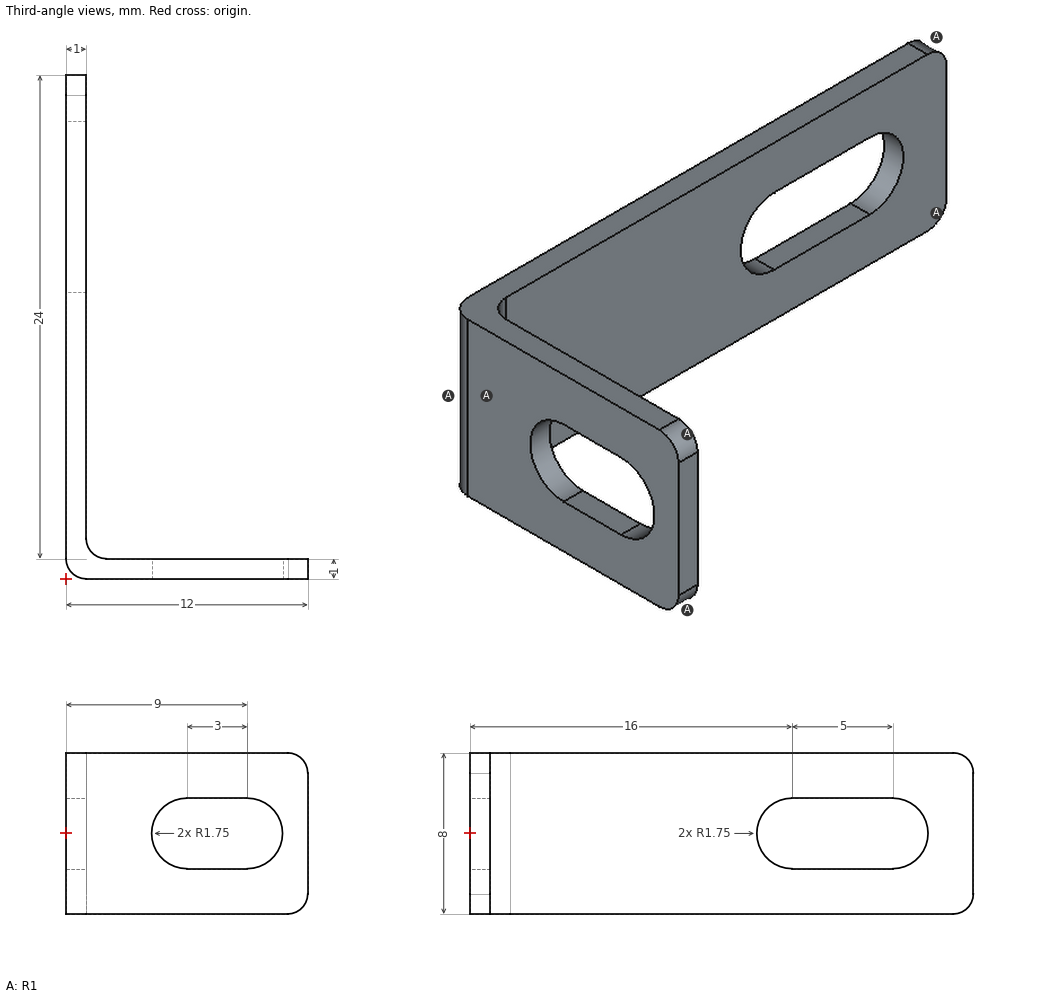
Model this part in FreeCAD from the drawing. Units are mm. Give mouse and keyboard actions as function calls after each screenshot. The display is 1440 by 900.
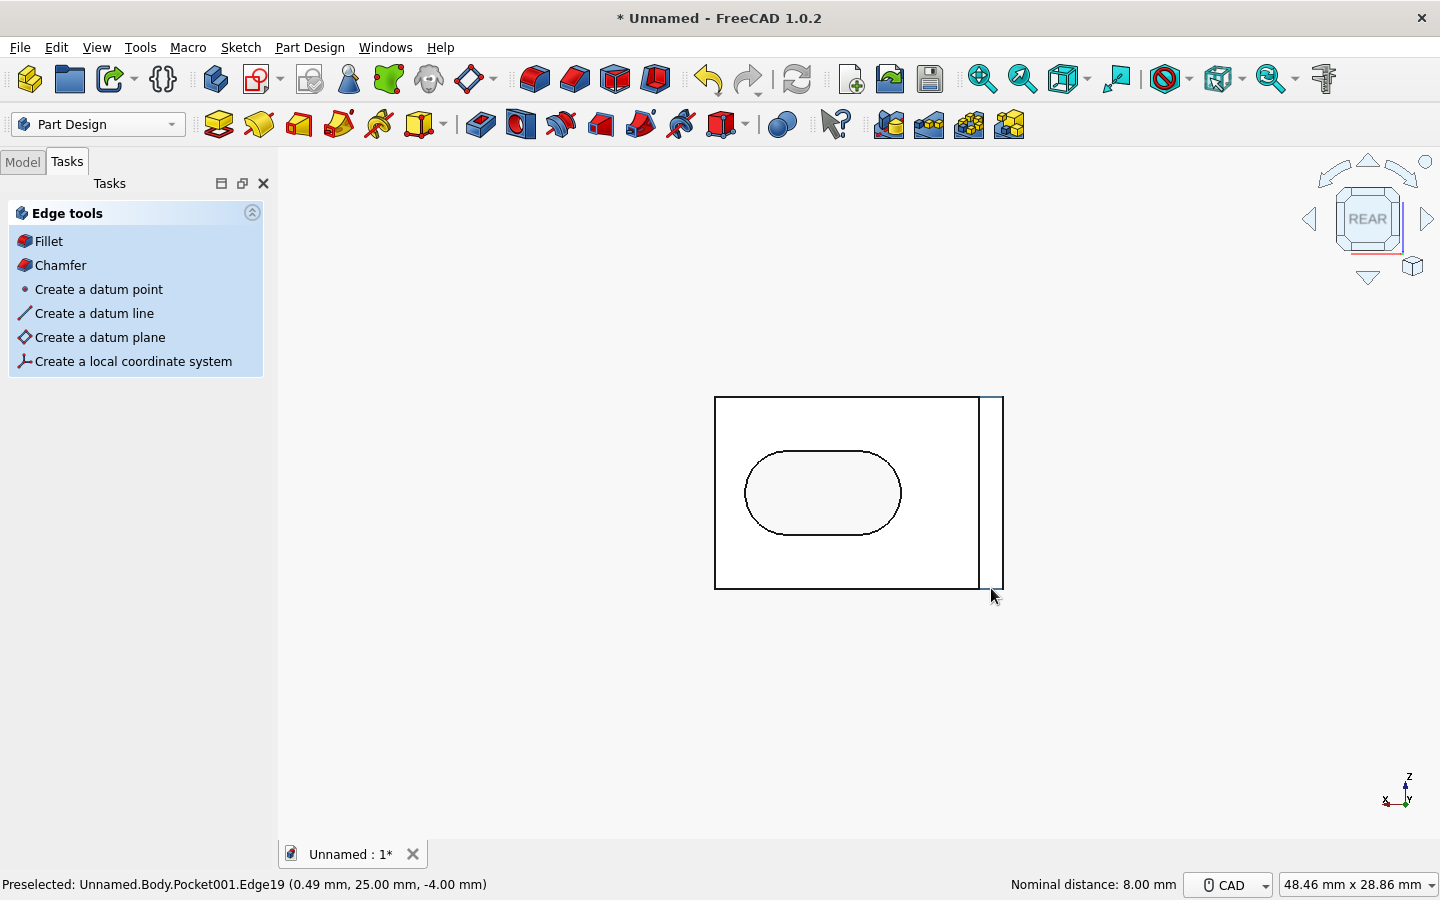
key(0)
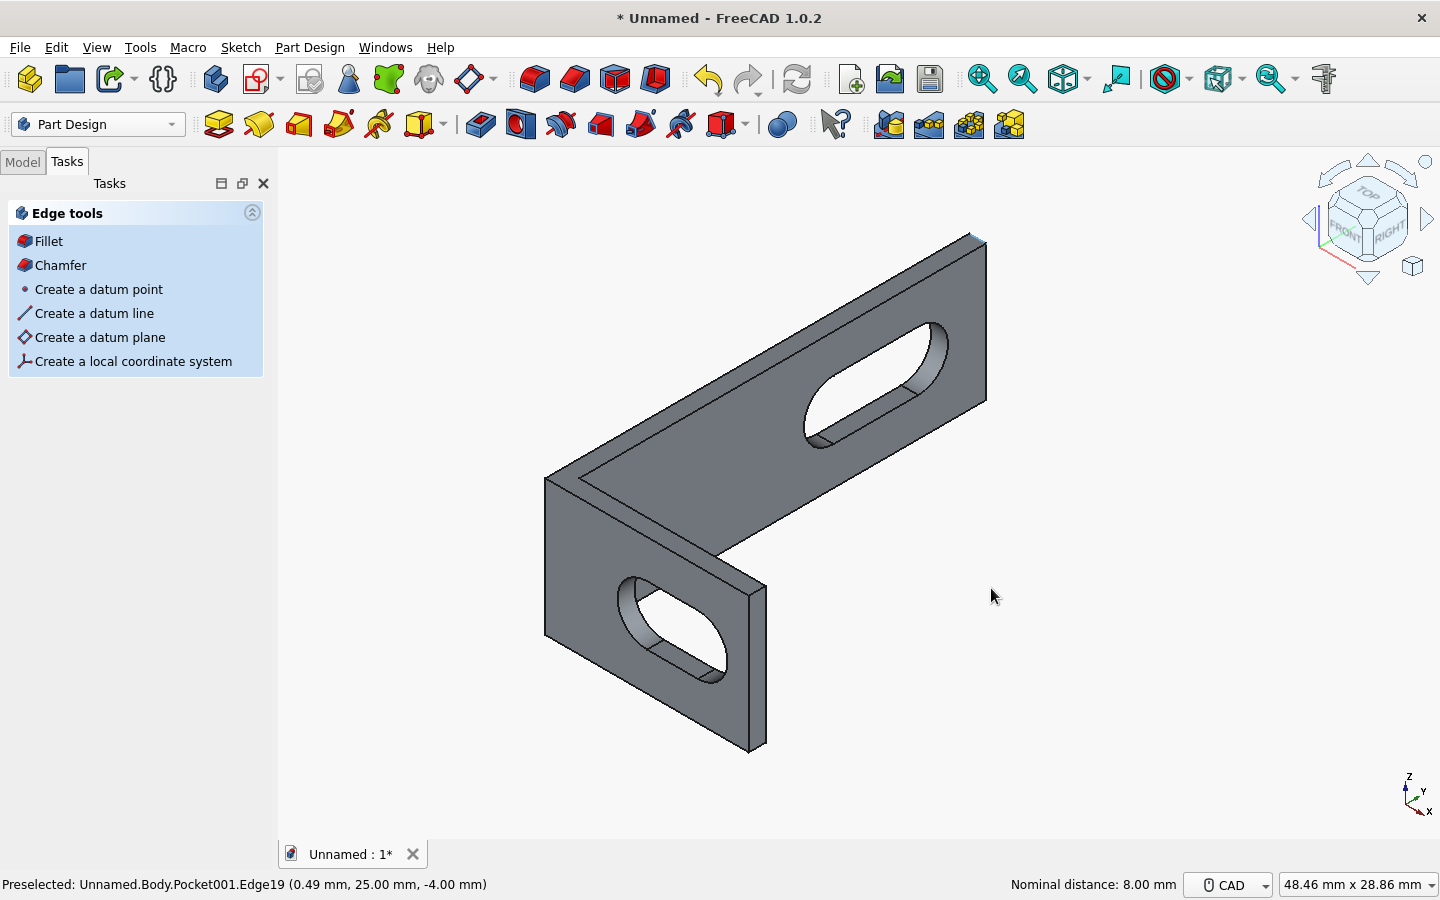
click(757, 590, ctrl)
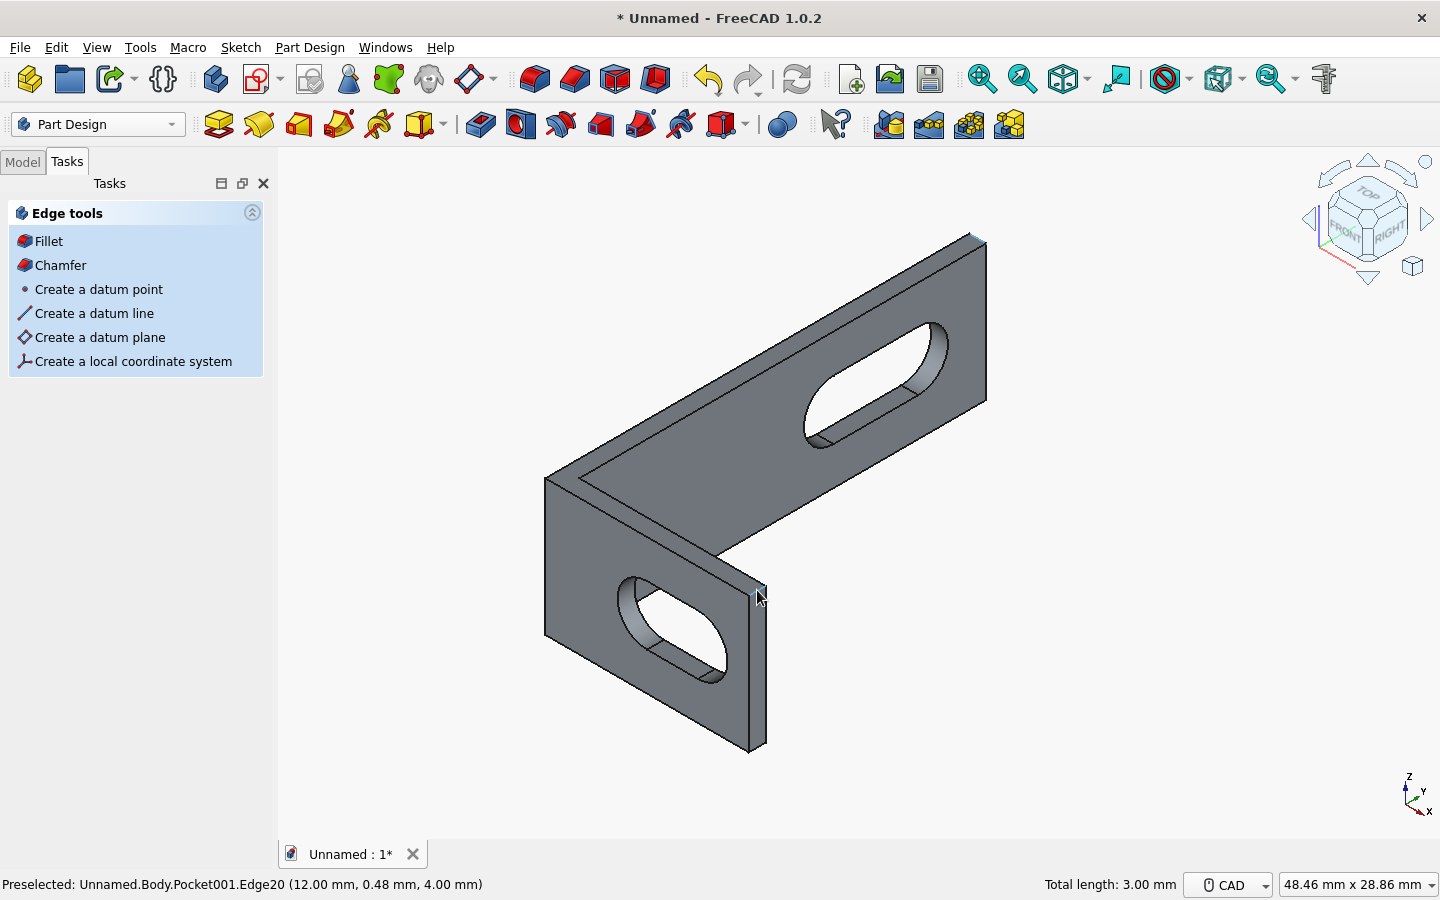
key(2)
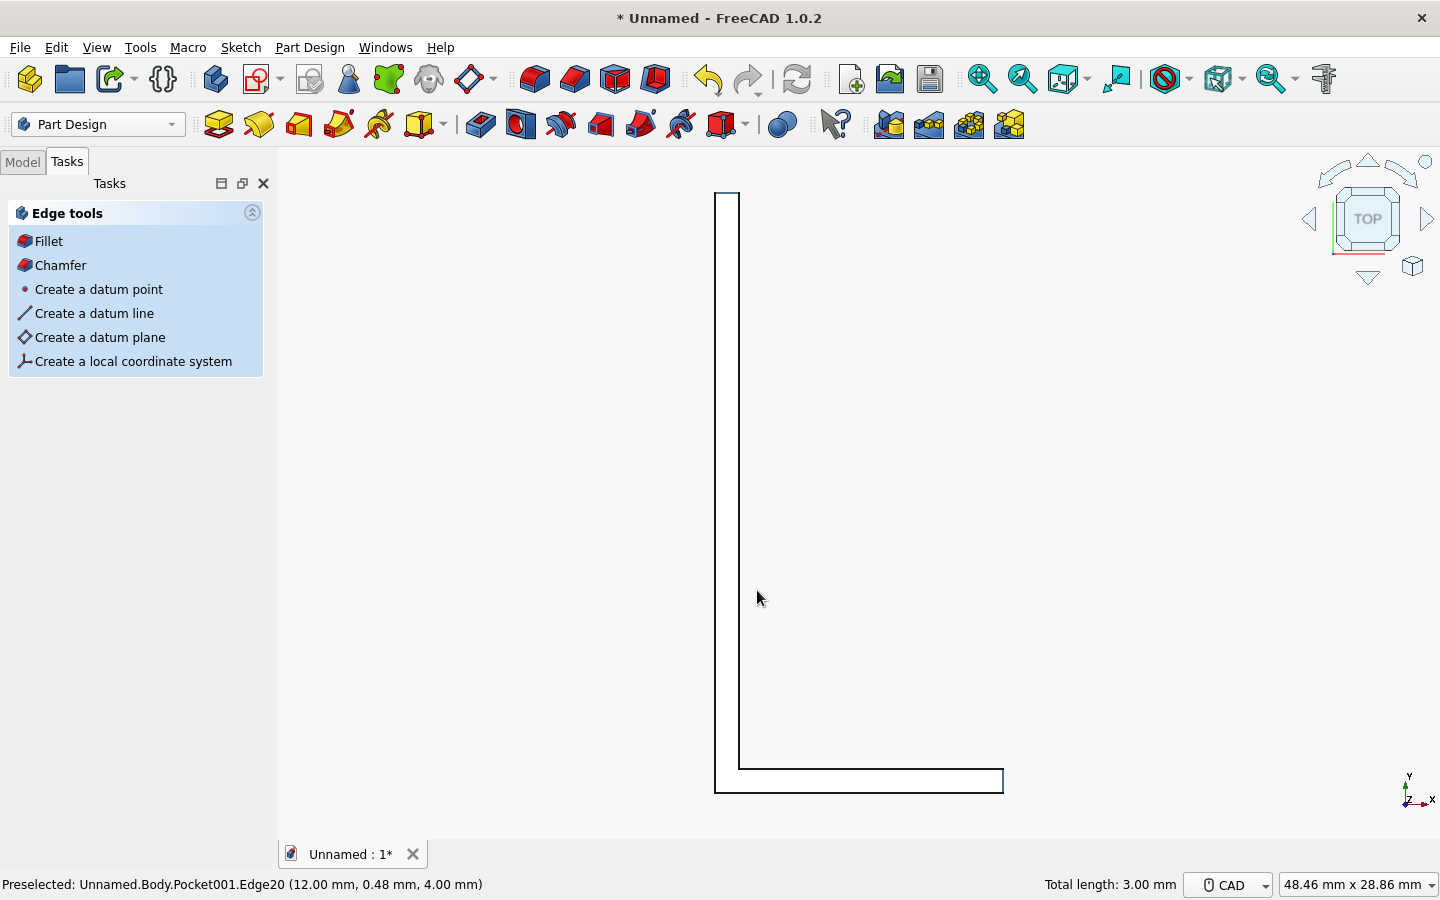
key(1)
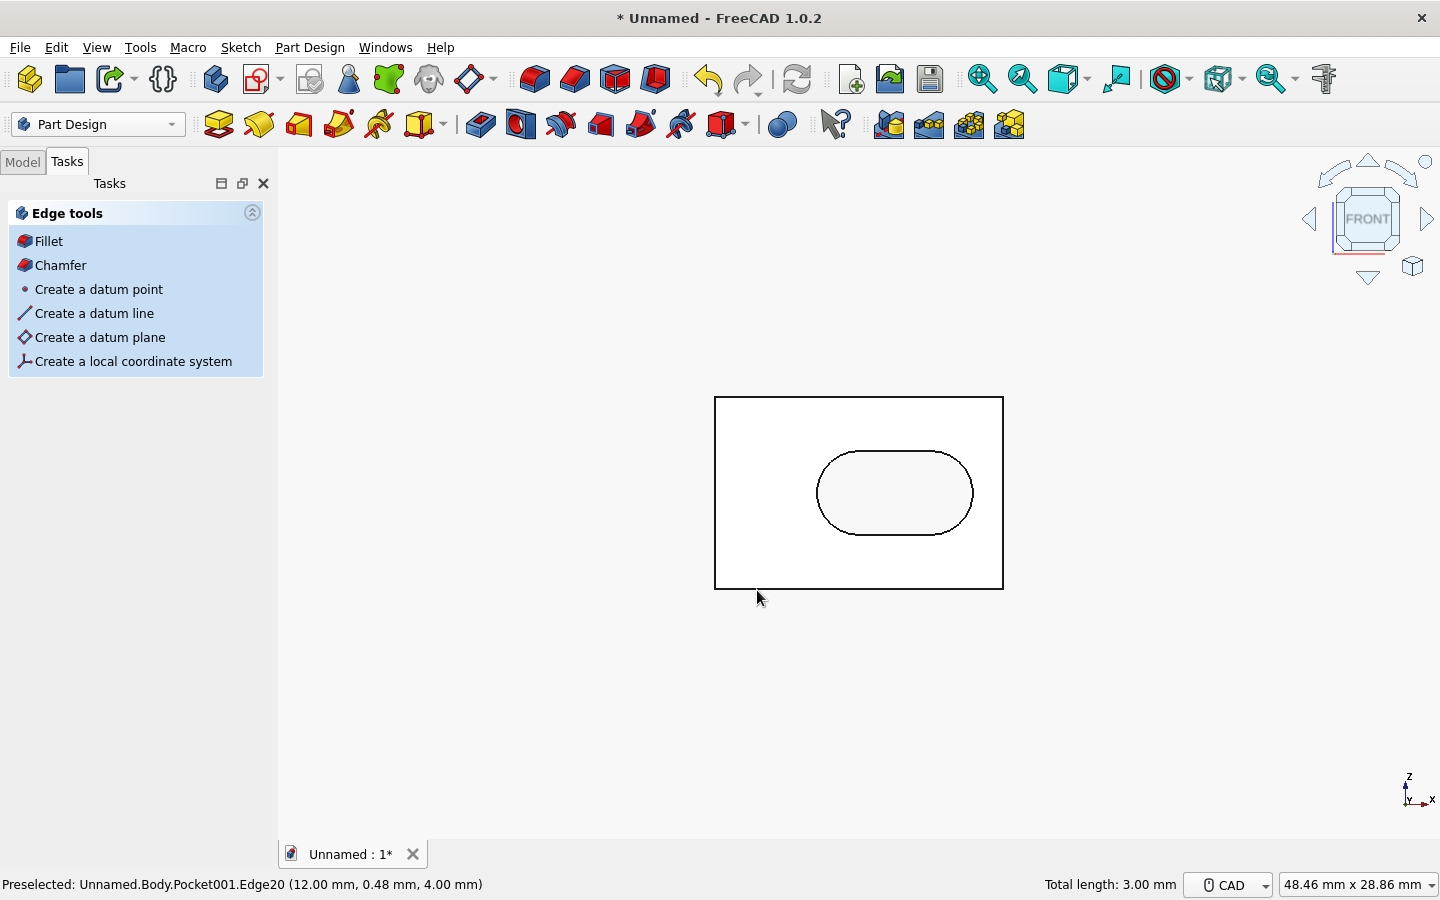
key(v)
key(f)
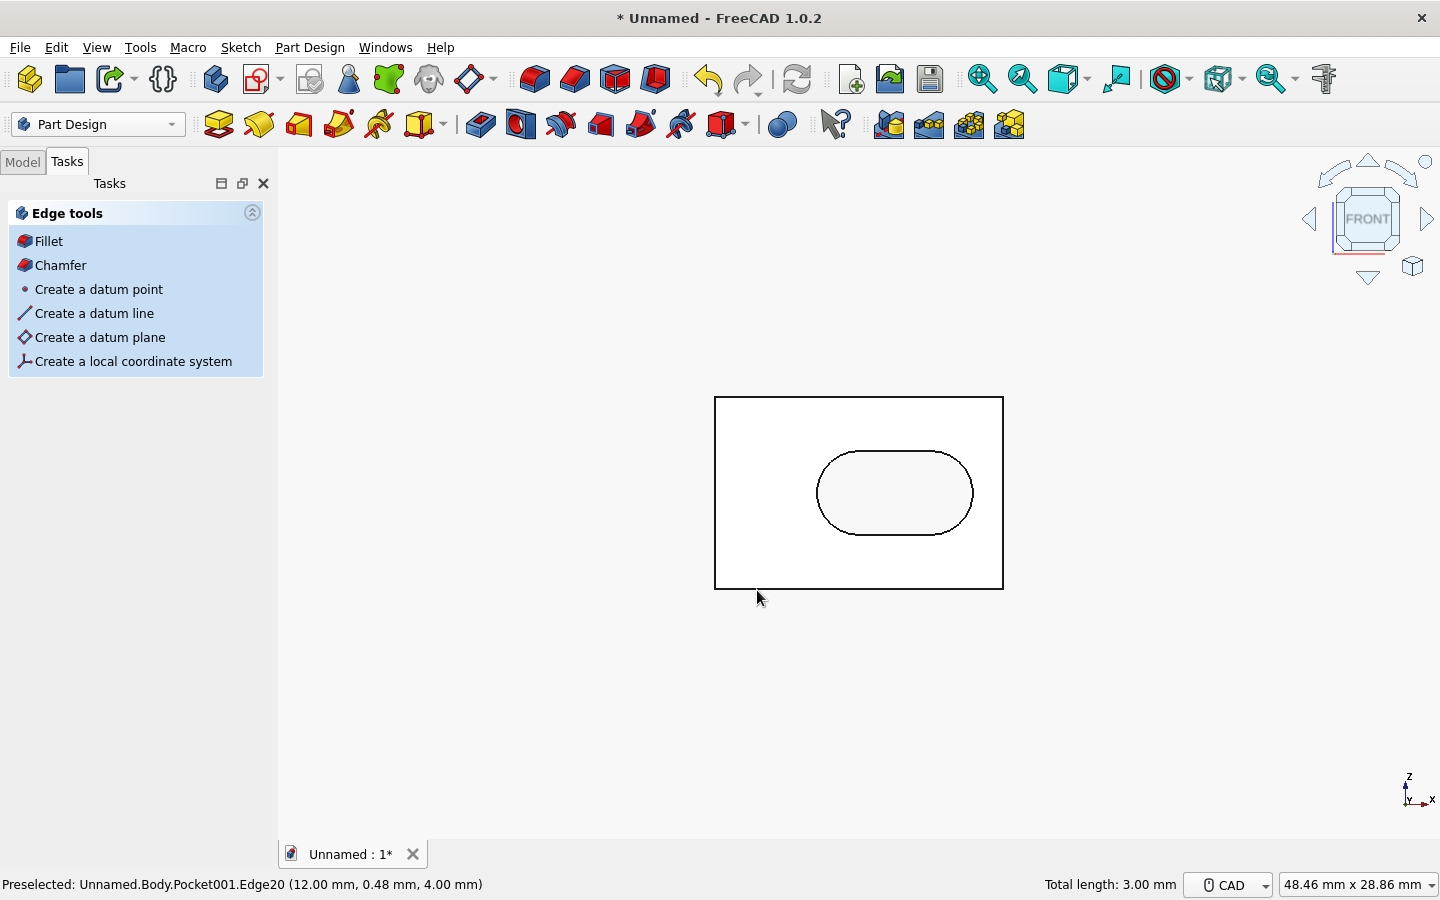
click(715, 492, ctrl)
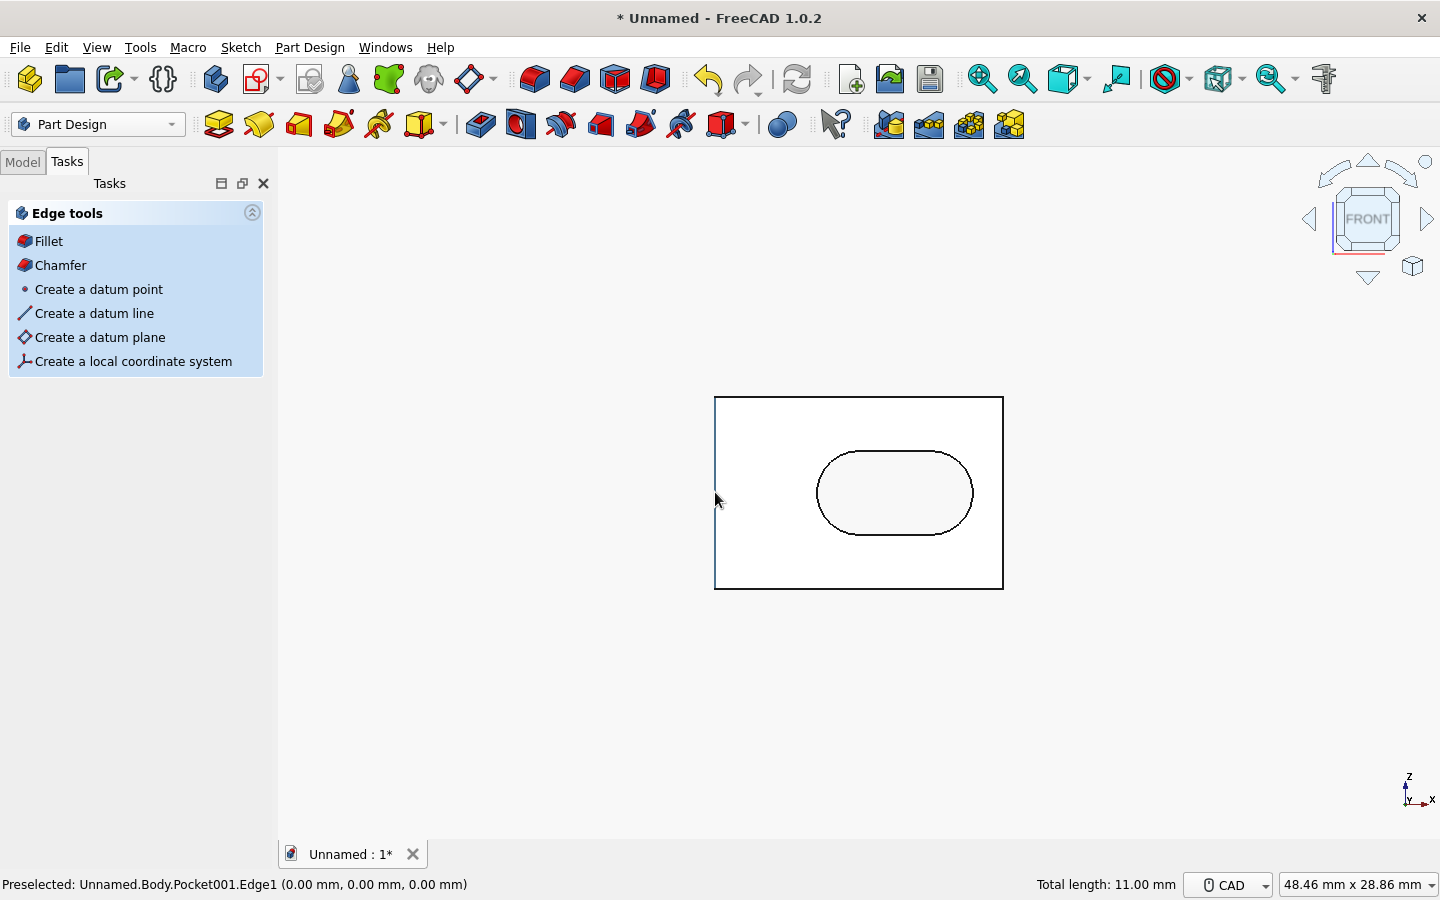
key(3)